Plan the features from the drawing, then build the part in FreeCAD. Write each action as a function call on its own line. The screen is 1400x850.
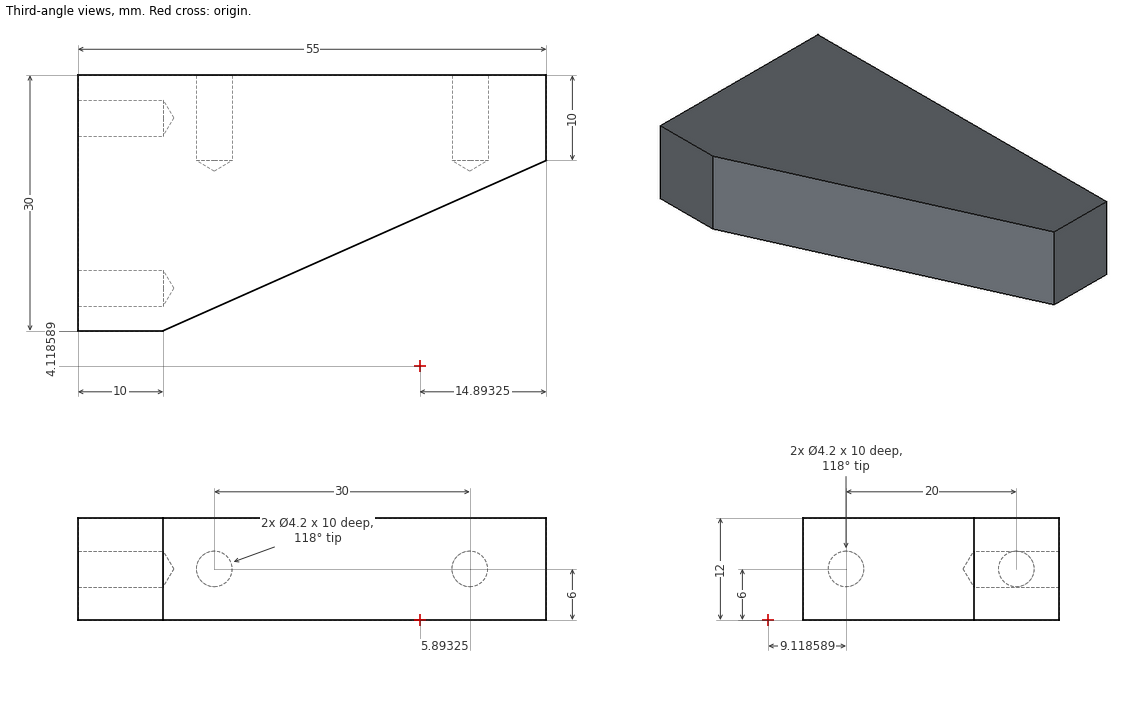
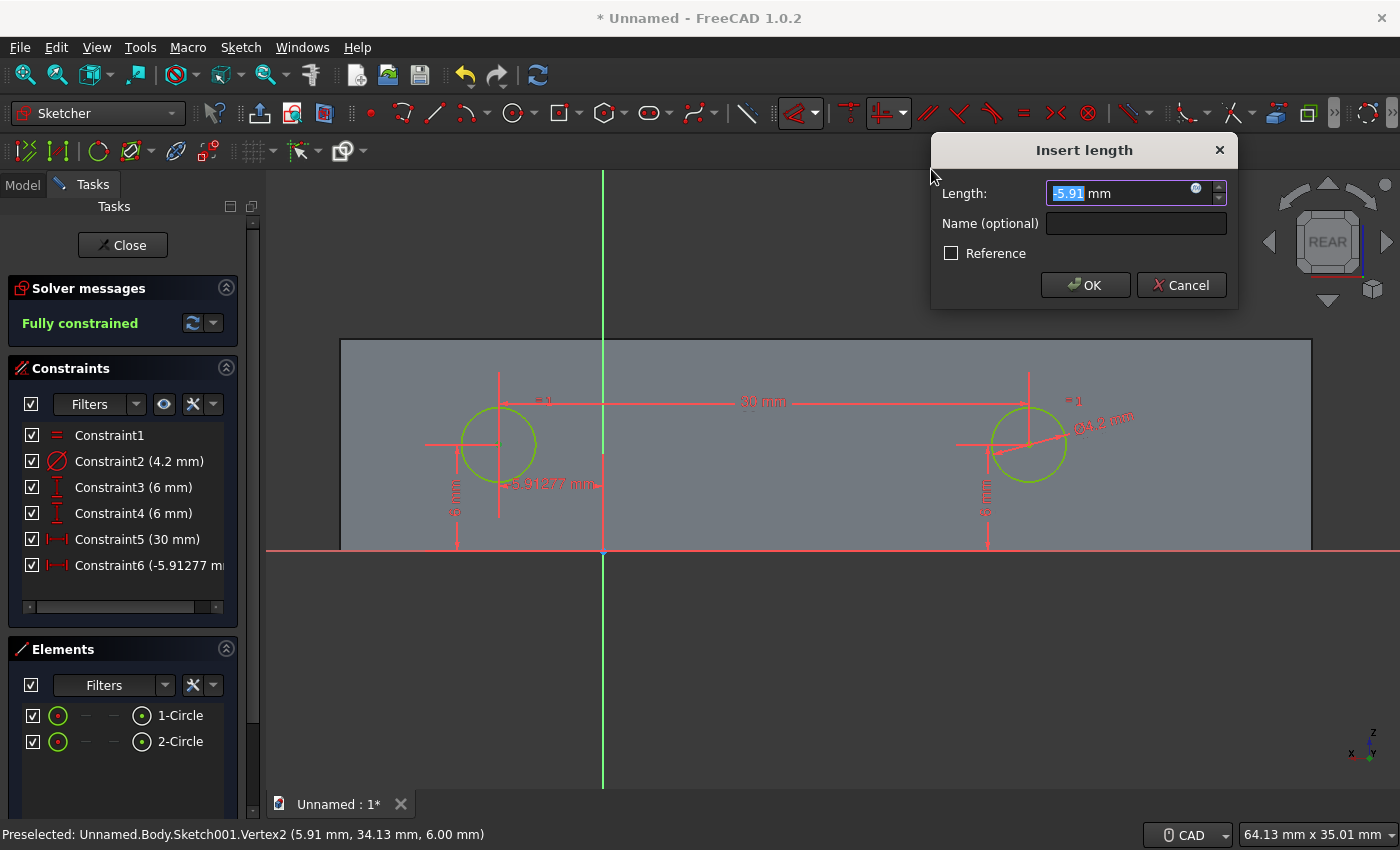
text(-5.89325)
key(Return)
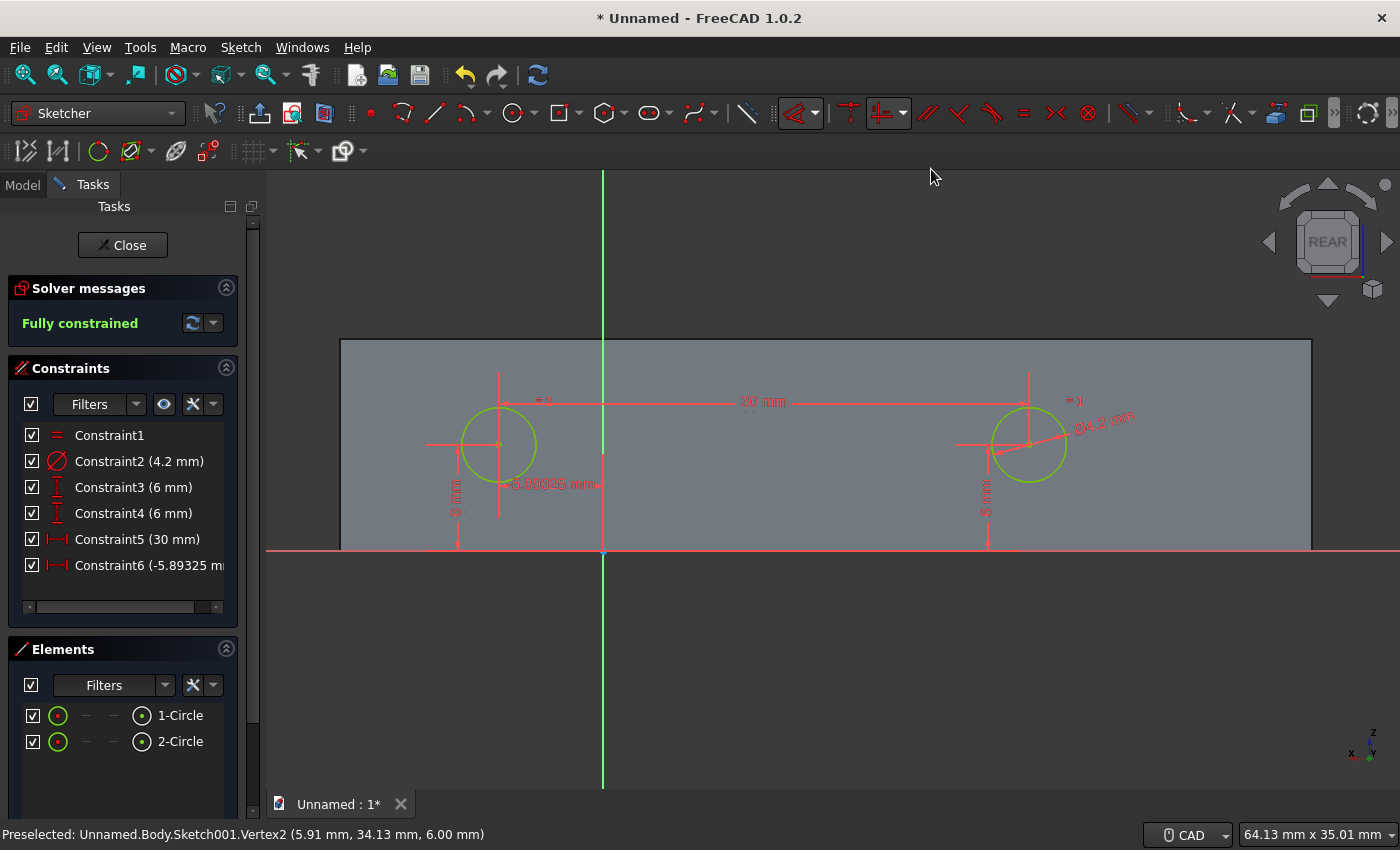
click(123, 245)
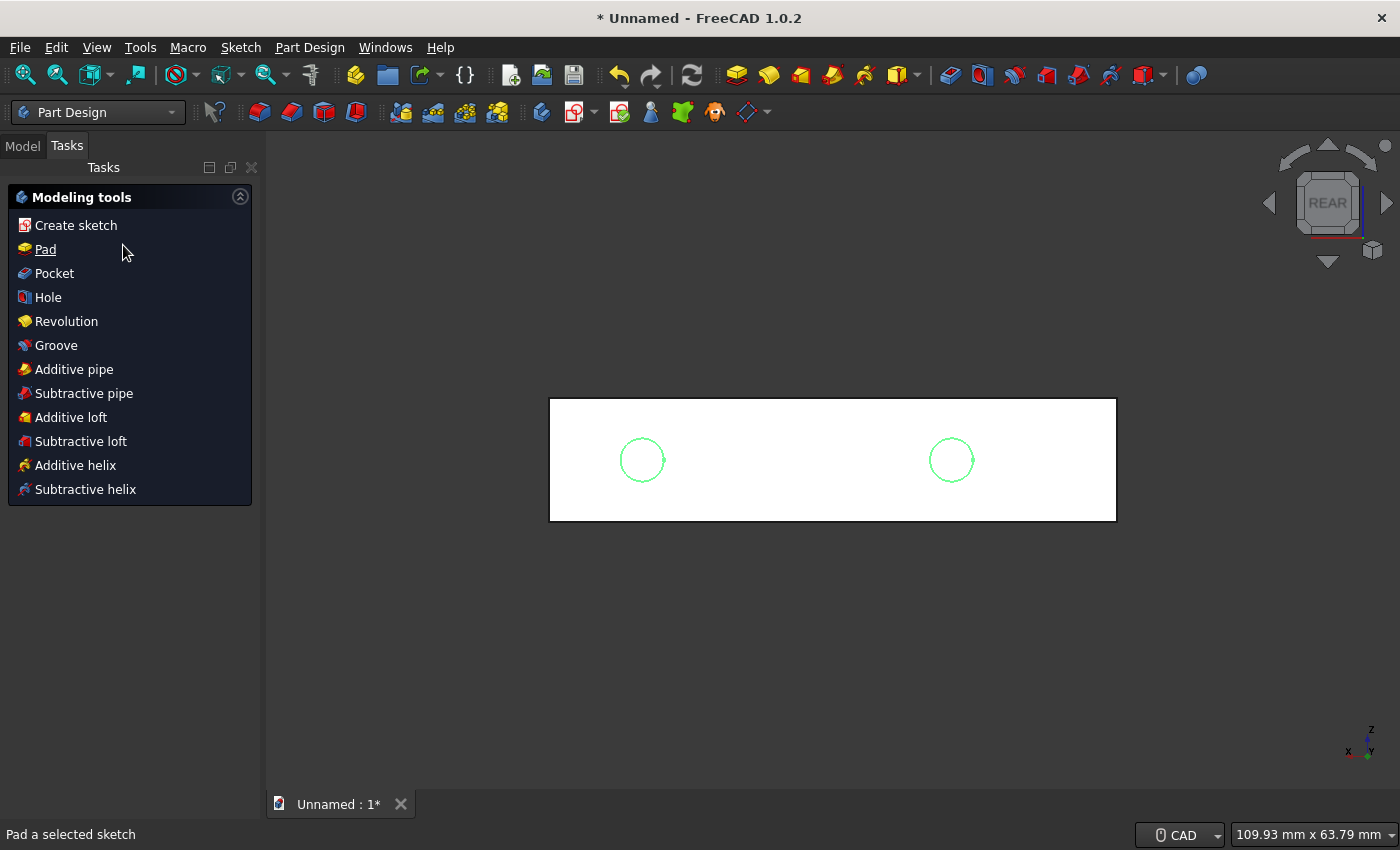
click(984, 76)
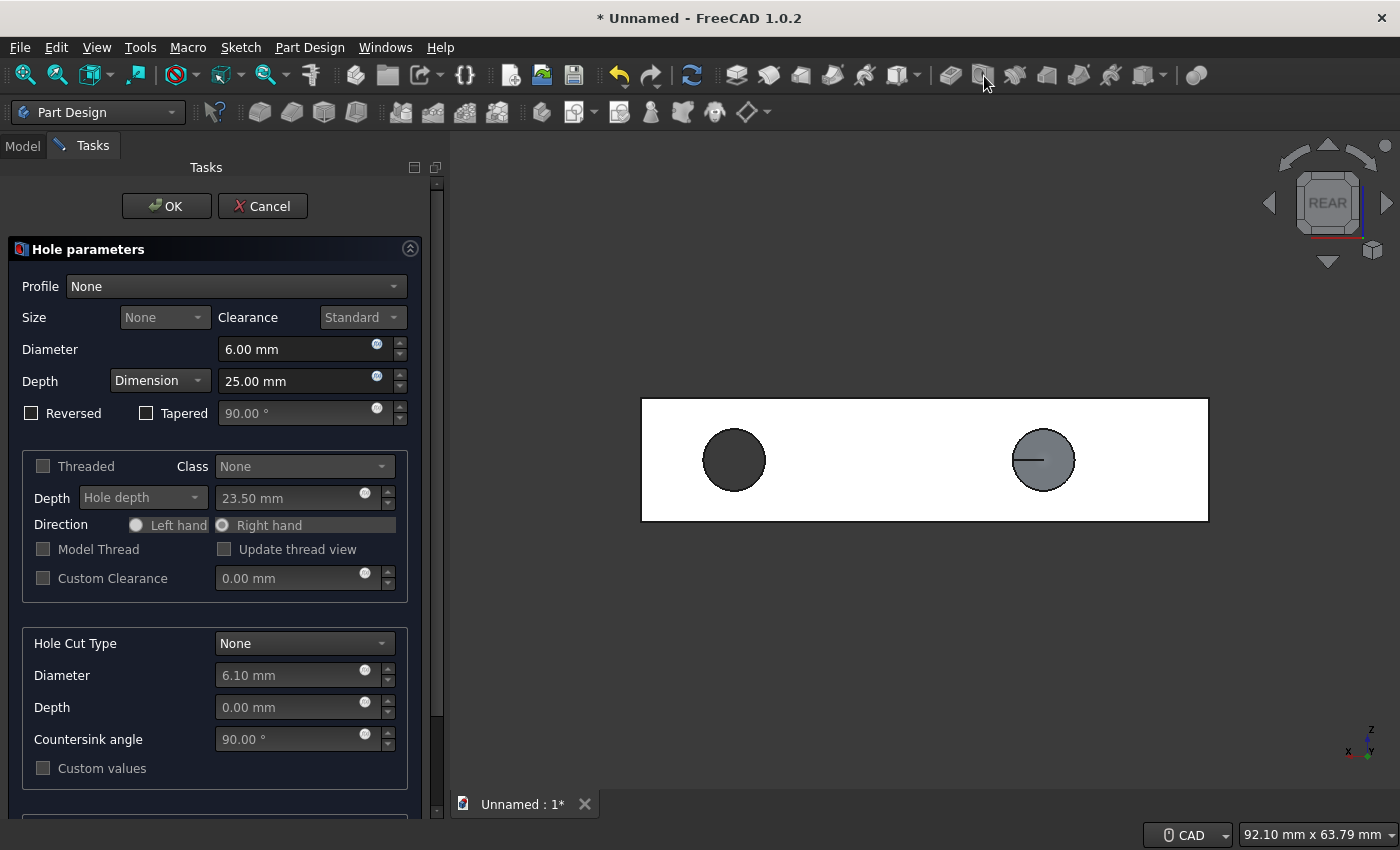
triple_click(305, 349)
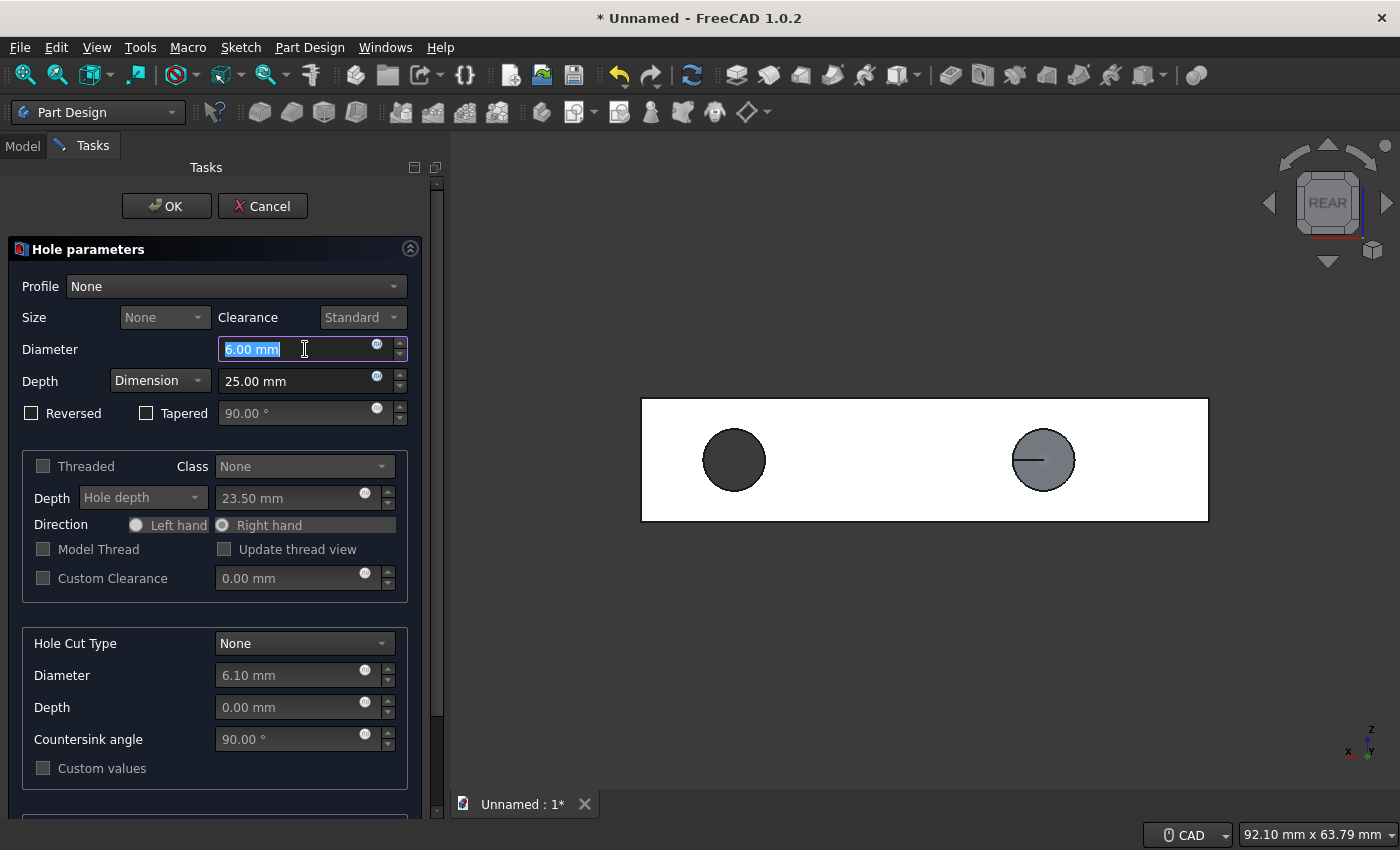
text(4.2)
key(Tab)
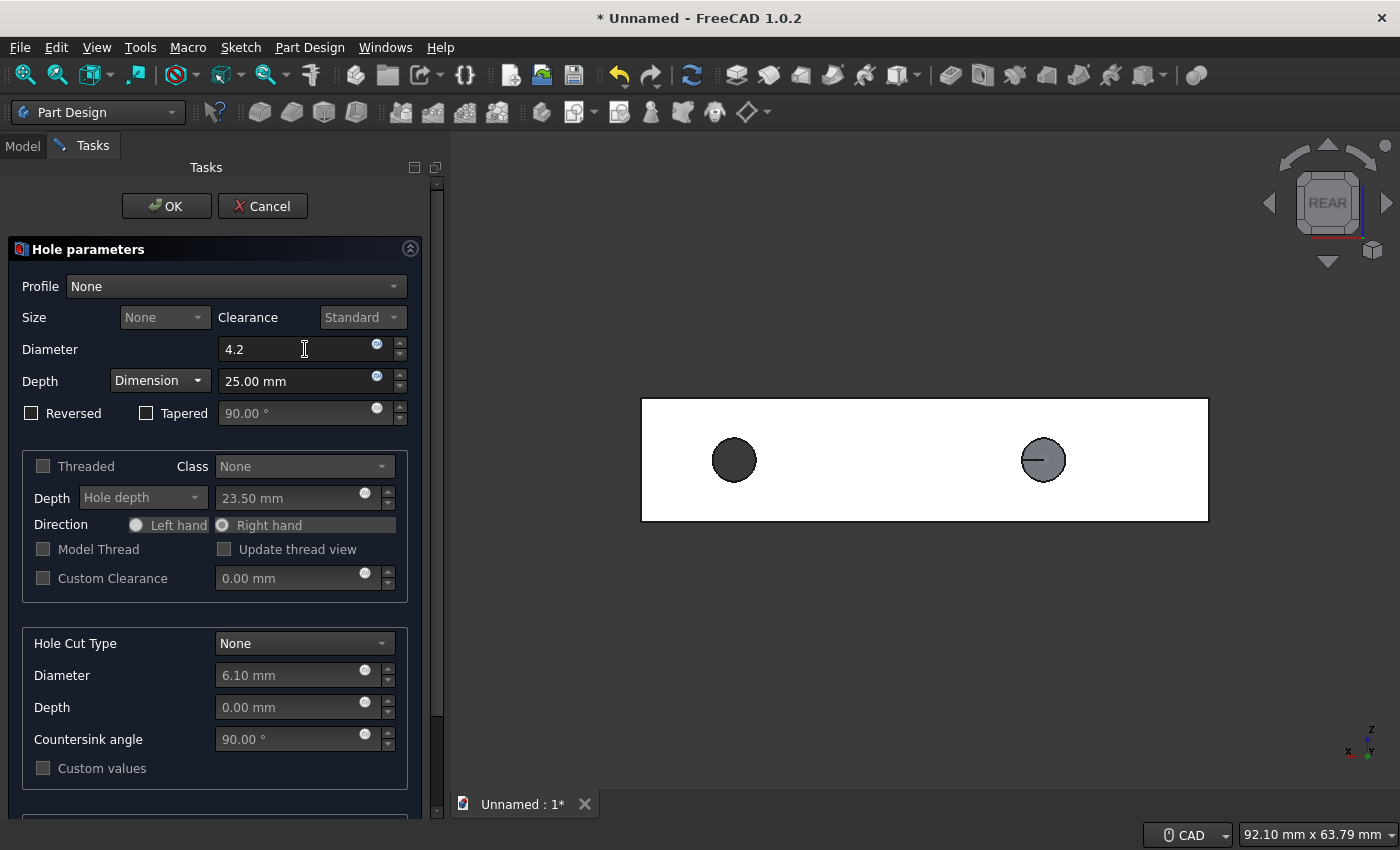
triple_click(305, 381)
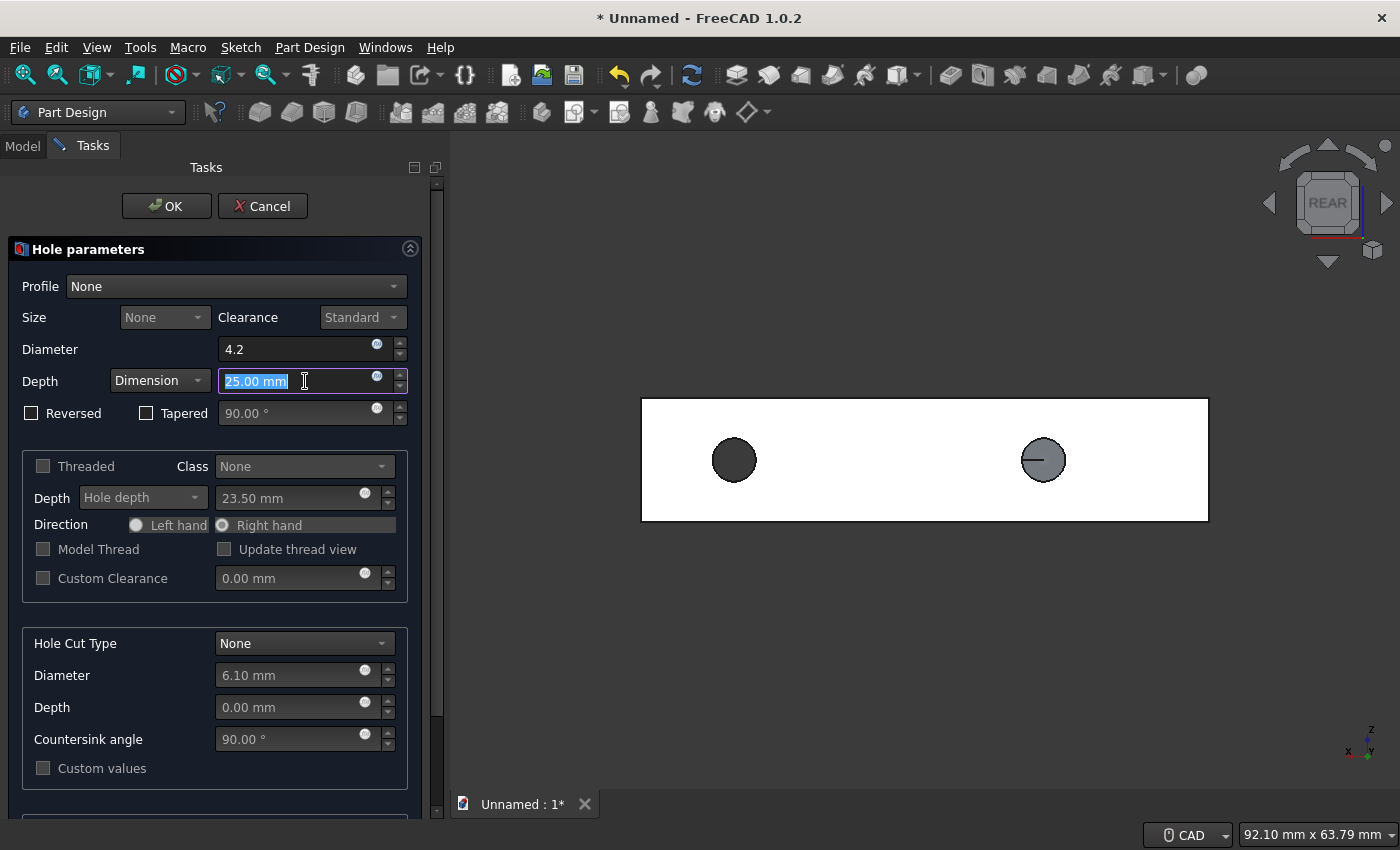
text(10)
key(Tab)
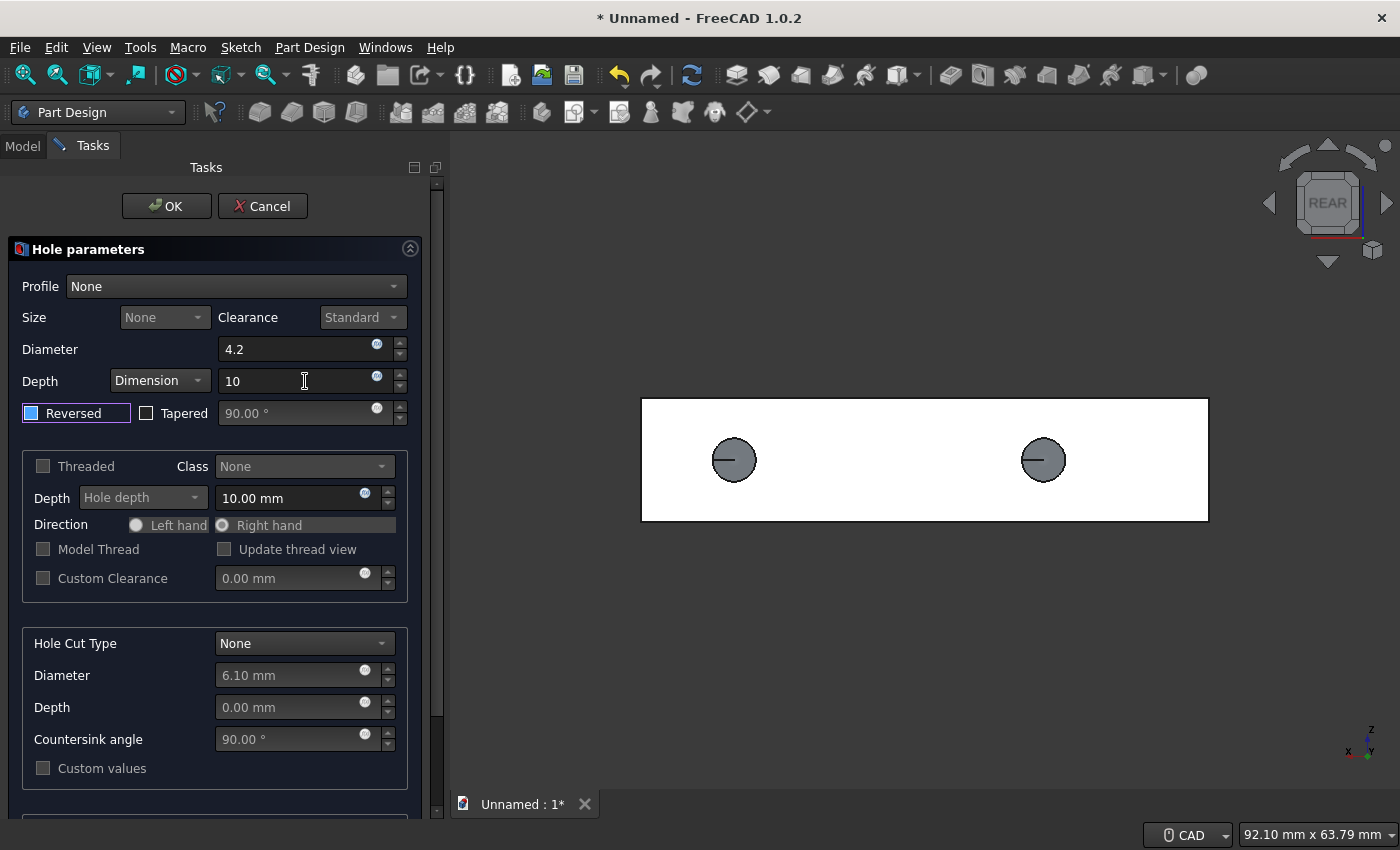
click(167, 206)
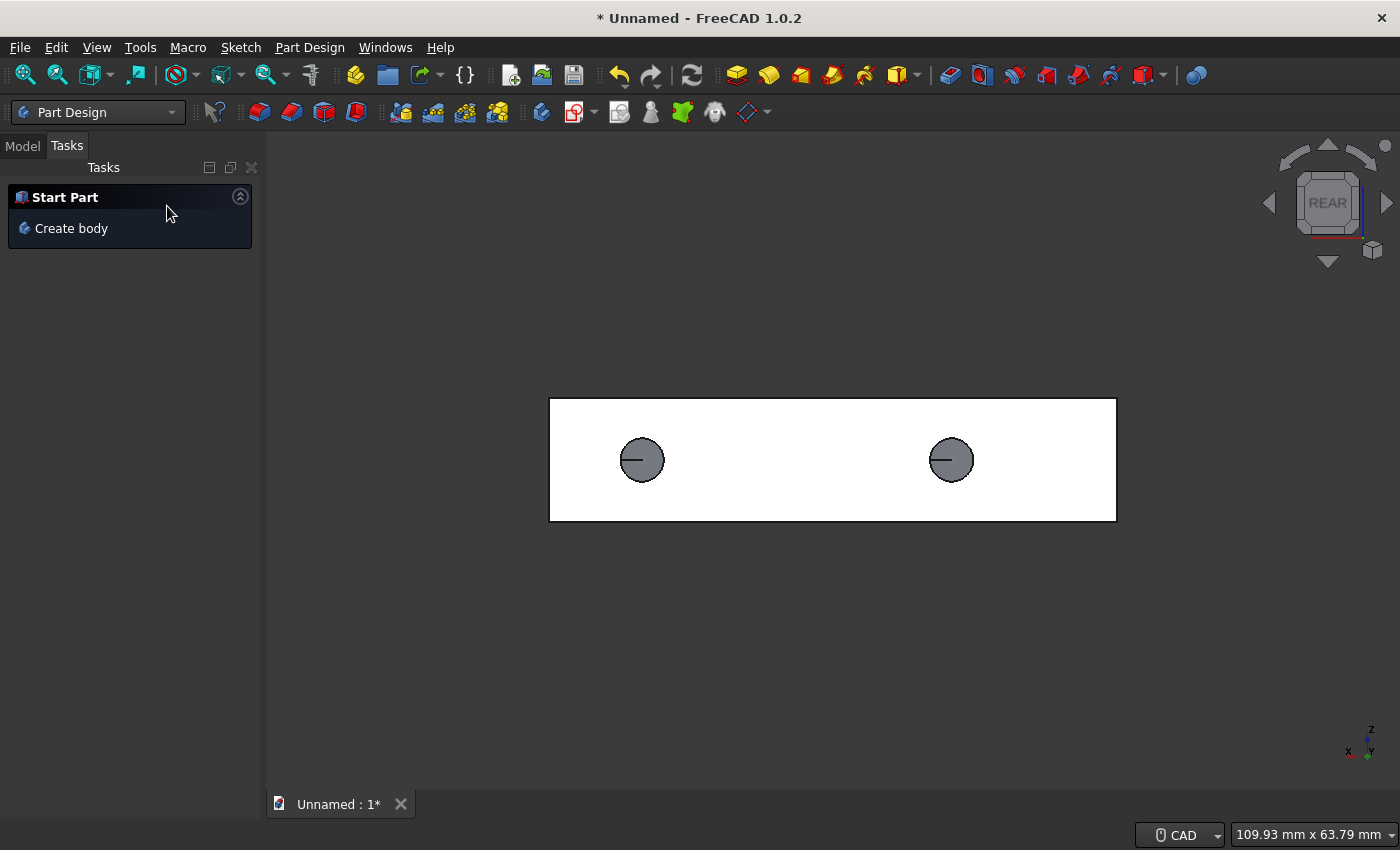
key(6)